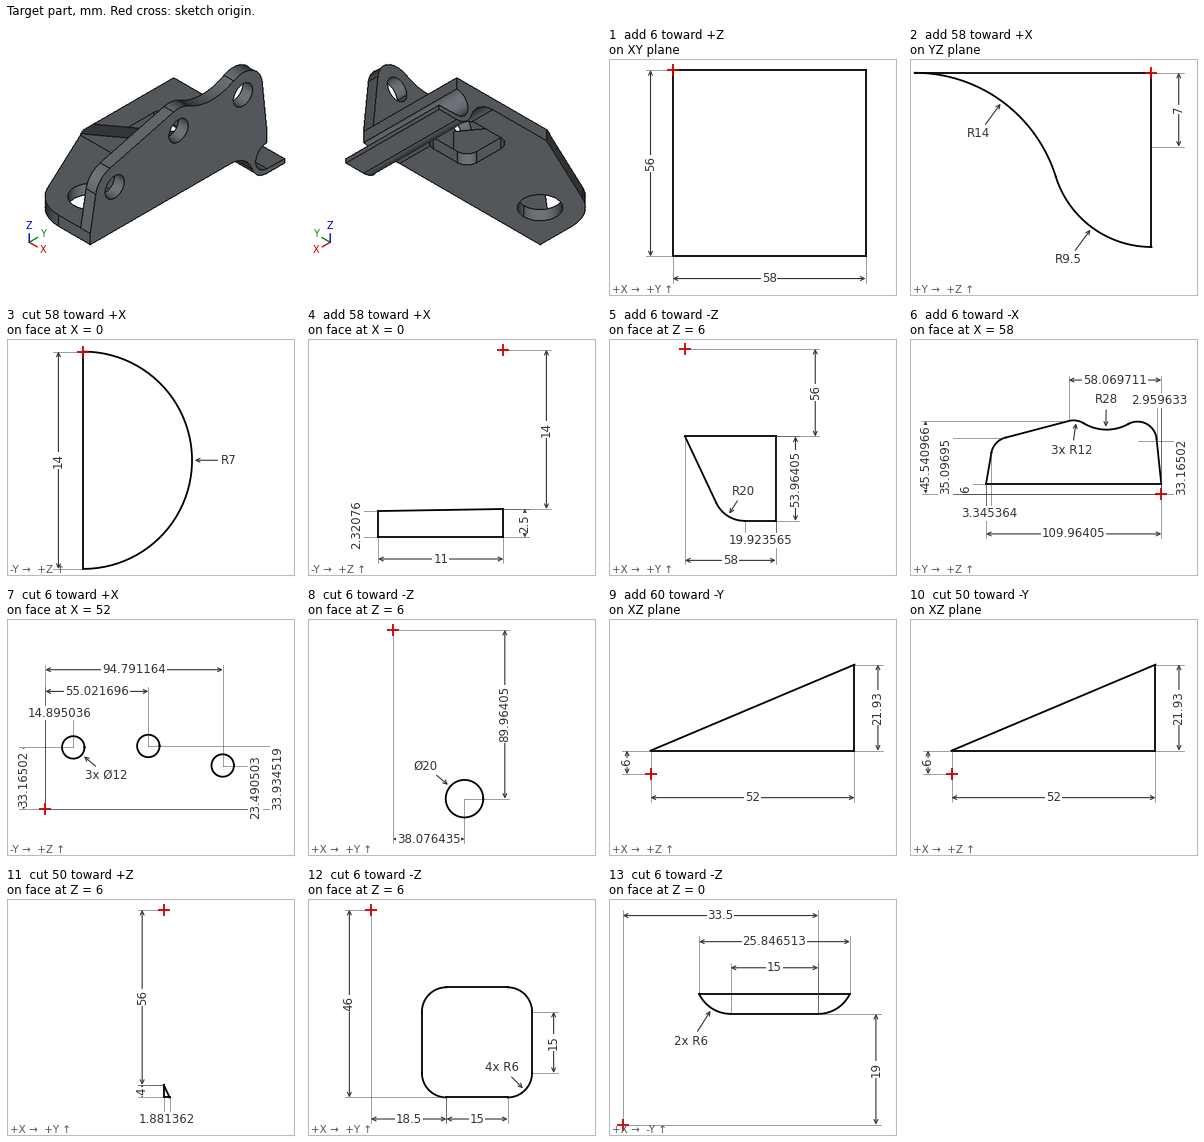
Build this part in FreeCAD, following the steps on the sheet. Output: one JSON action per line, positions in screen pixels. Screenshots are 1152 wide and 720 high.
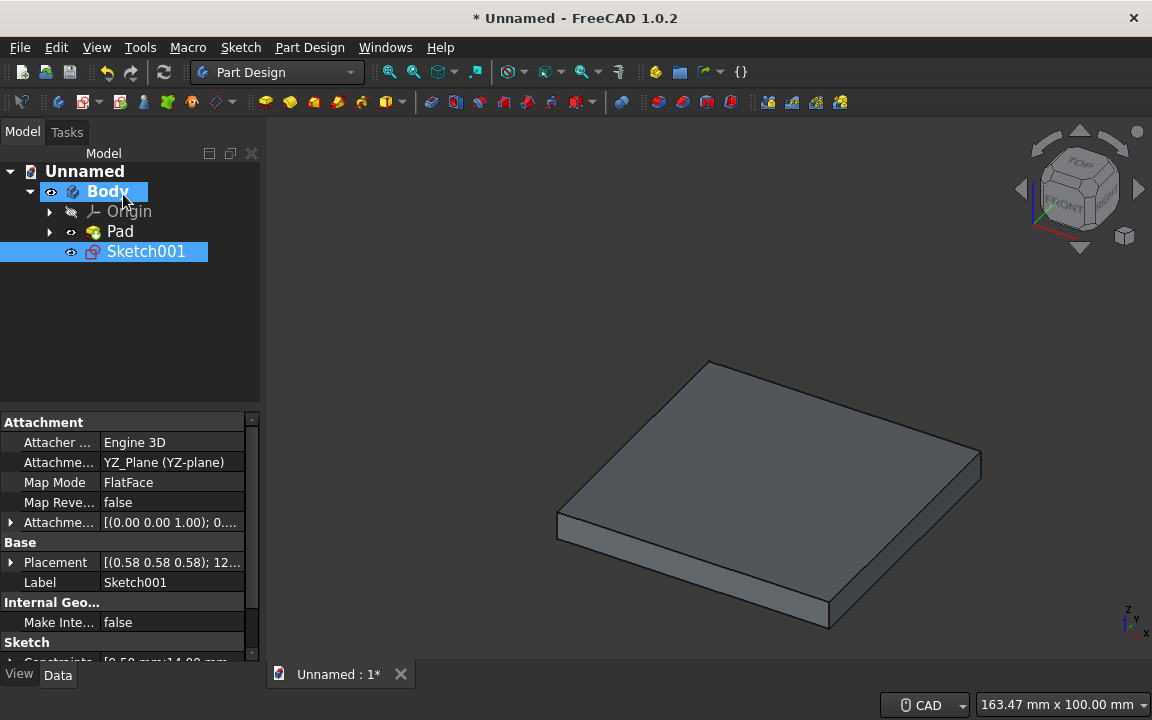
{"action": "left_click", "coordinate": [266, 102]}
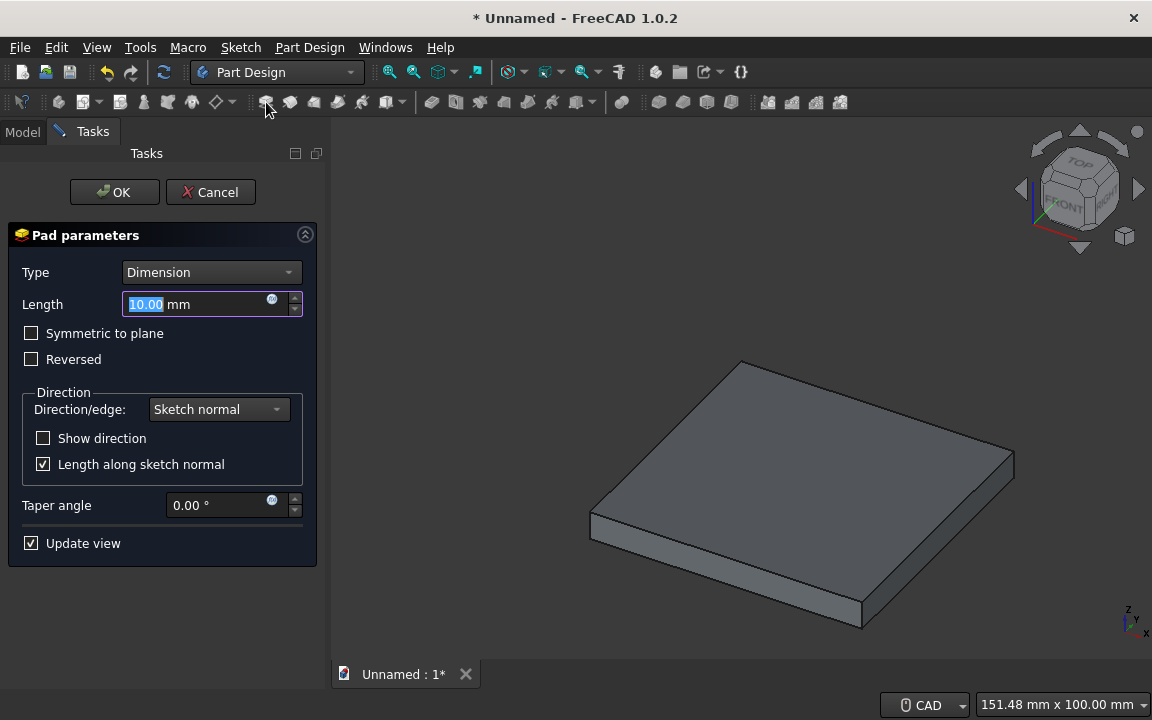
{"action": "type", "text": "58"}
{"action": "key", "text": "Tab"}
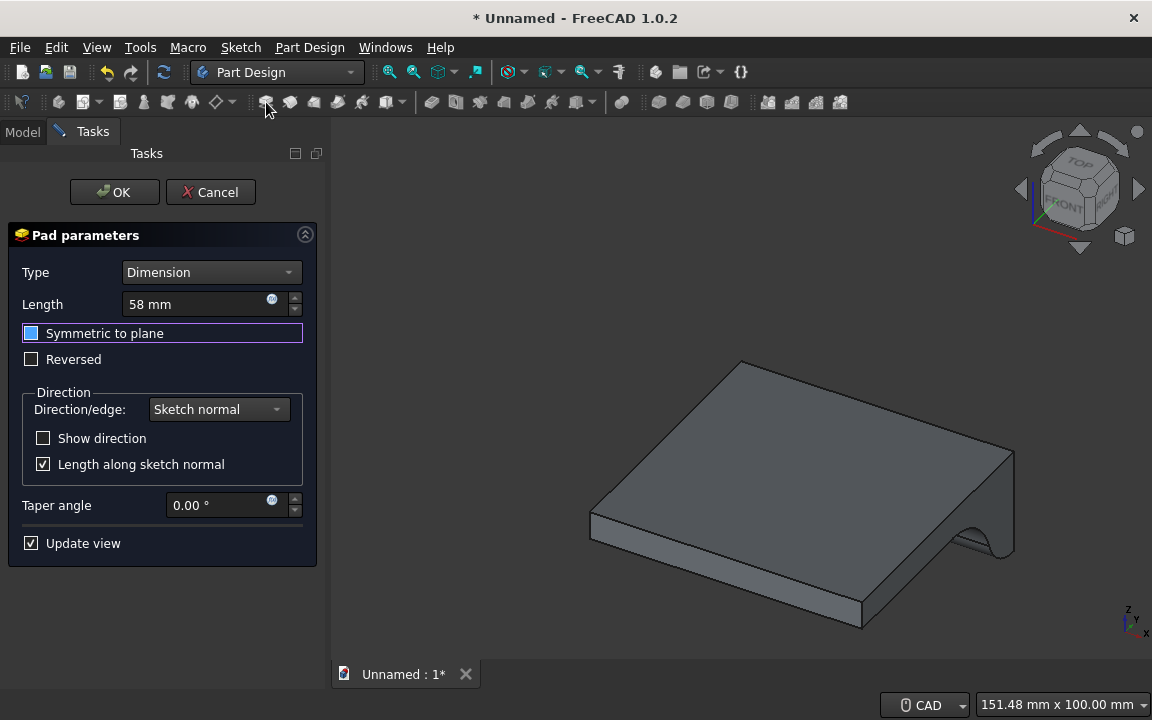
{"action": "left_click", "coordinate": [115, 192]}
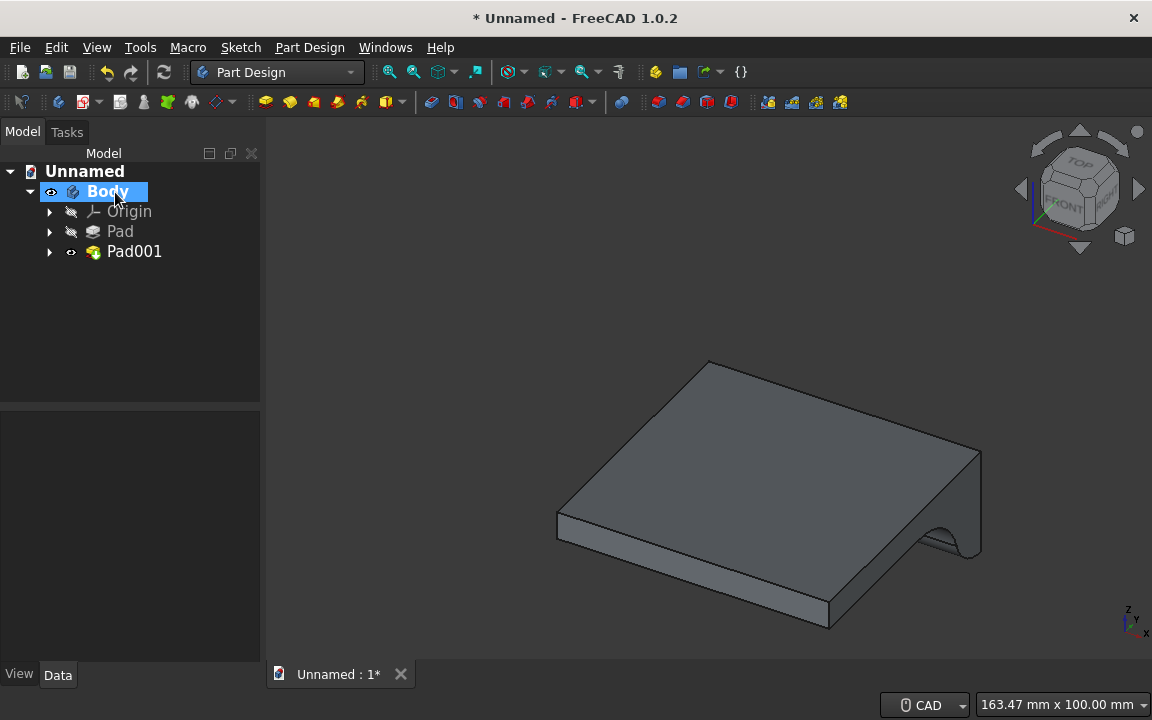
{"action": "left_click", "coordinate": [390, 72]}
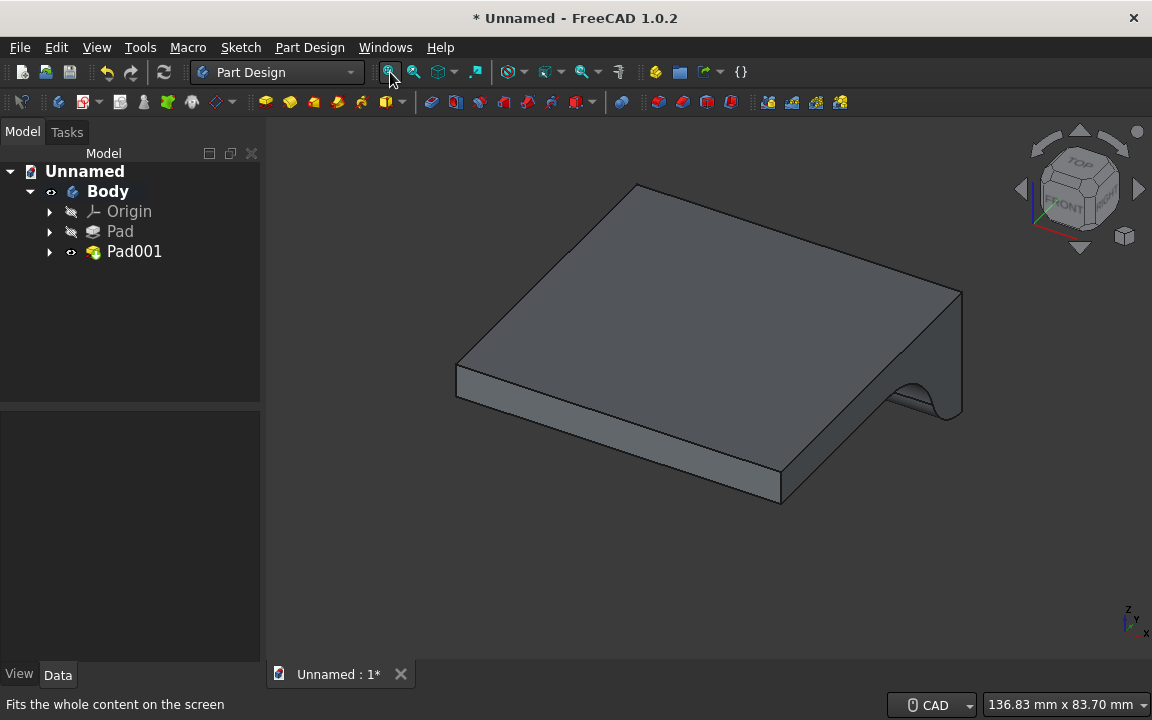
{"action": "key", "text": "6"}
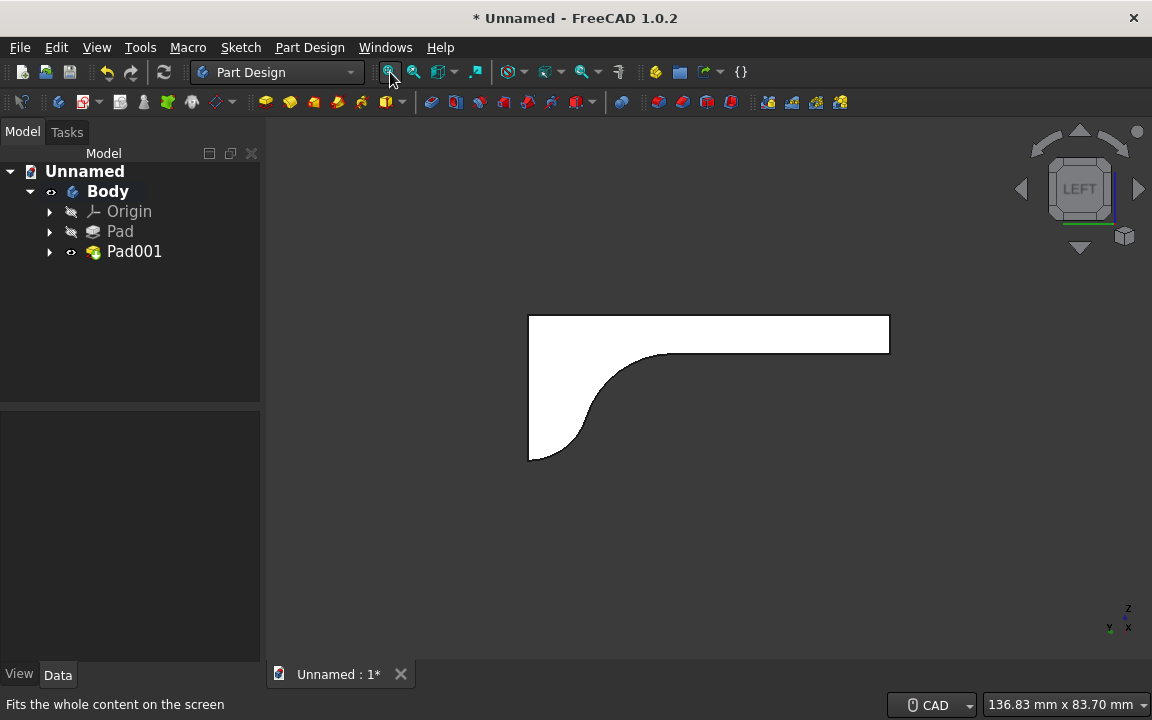
{"action": "left_click", "coordinate": [390, 72]}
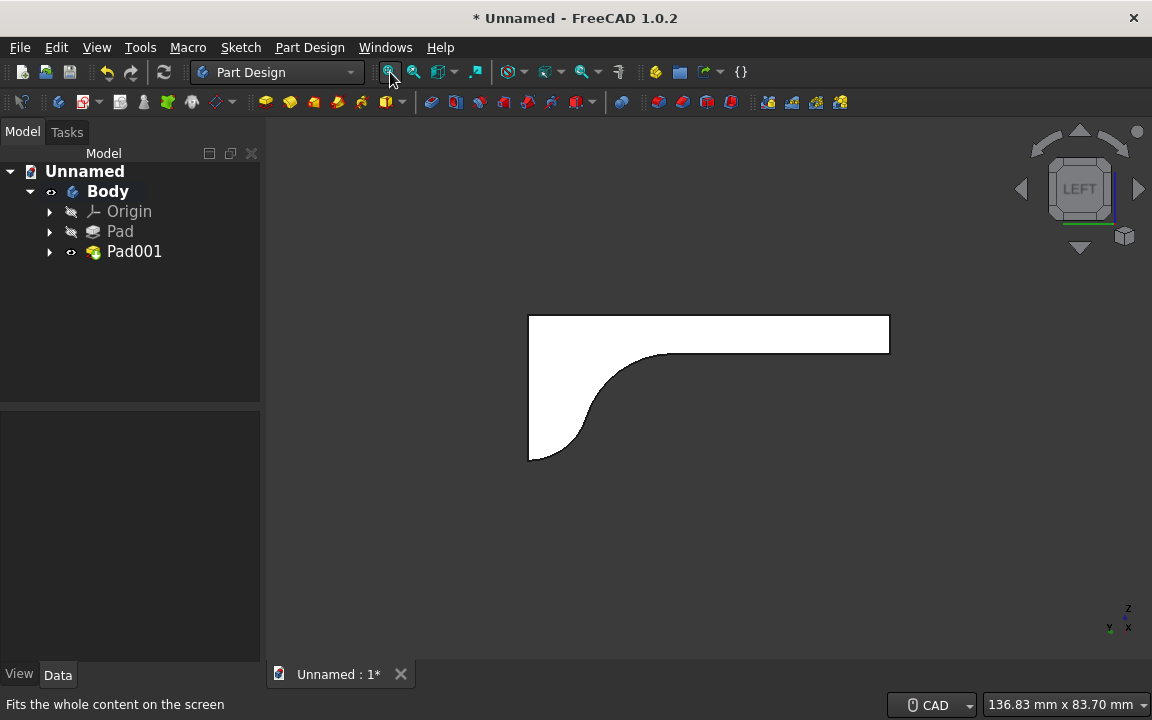
{"action": "left_click", "coordinate": [605, 345]}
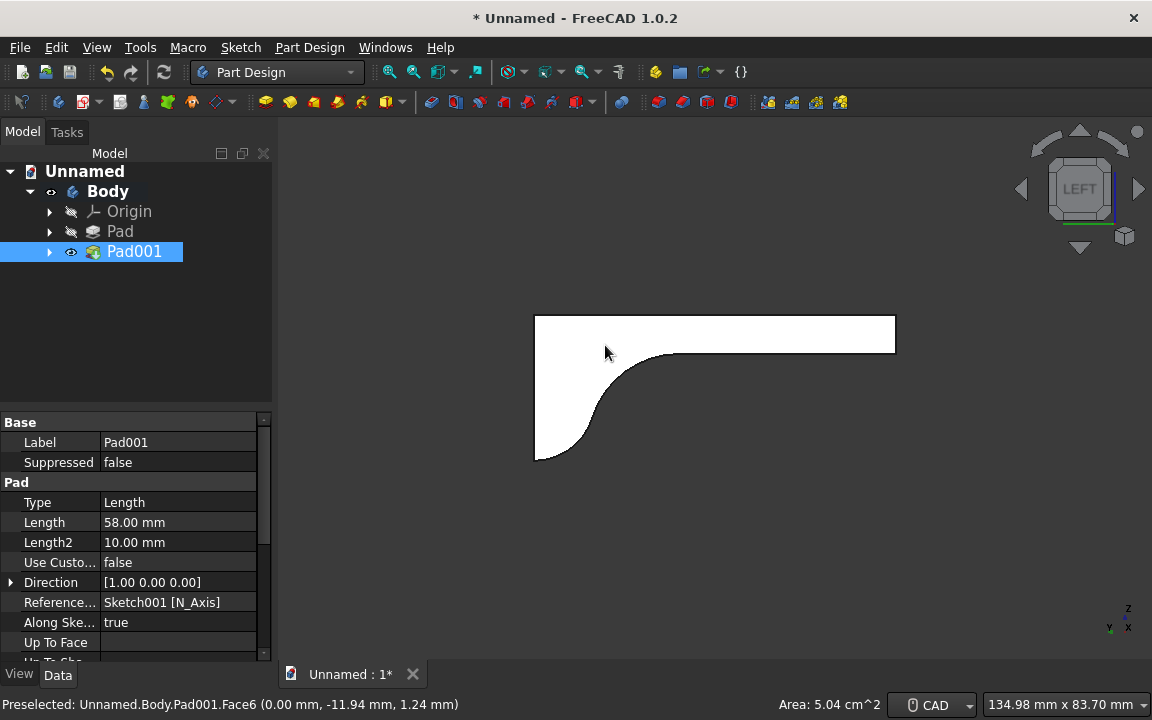
{"action": "left_click", "coordinate": [84, 102]}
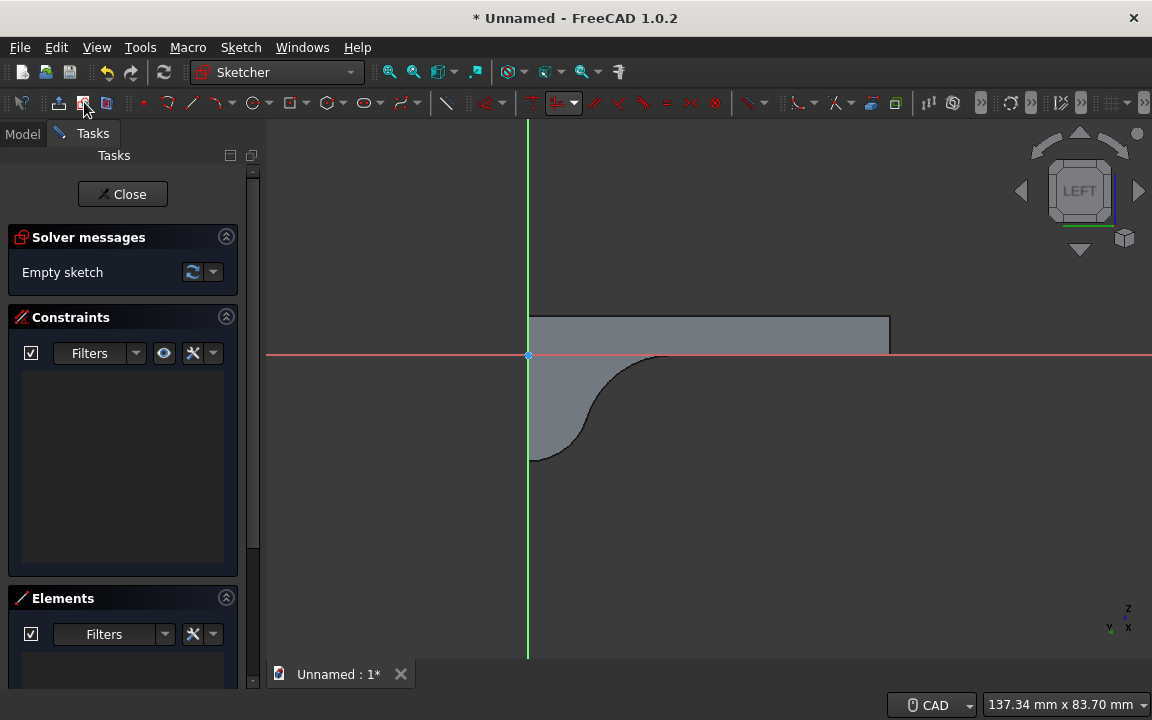
{"action": "scroll", "coordinate": [522, 404], "scroll_direction": "up", "scroll_amount": 7}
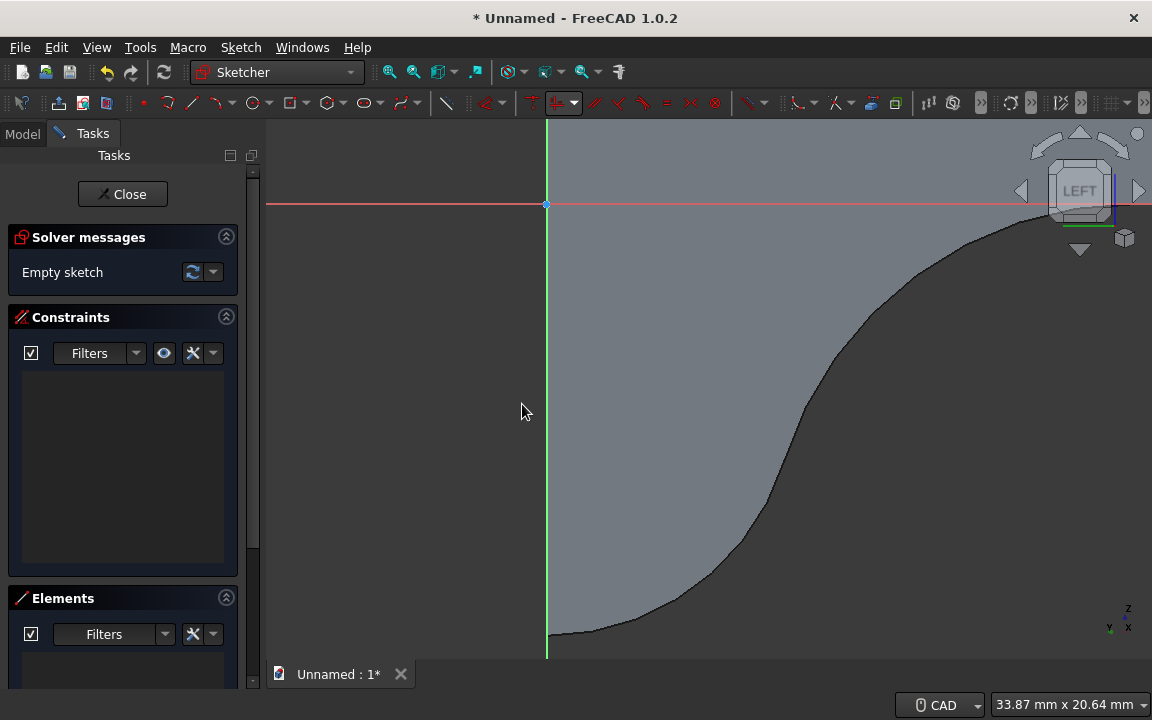
{"action": "left_click", "coordinate": [192, 104]}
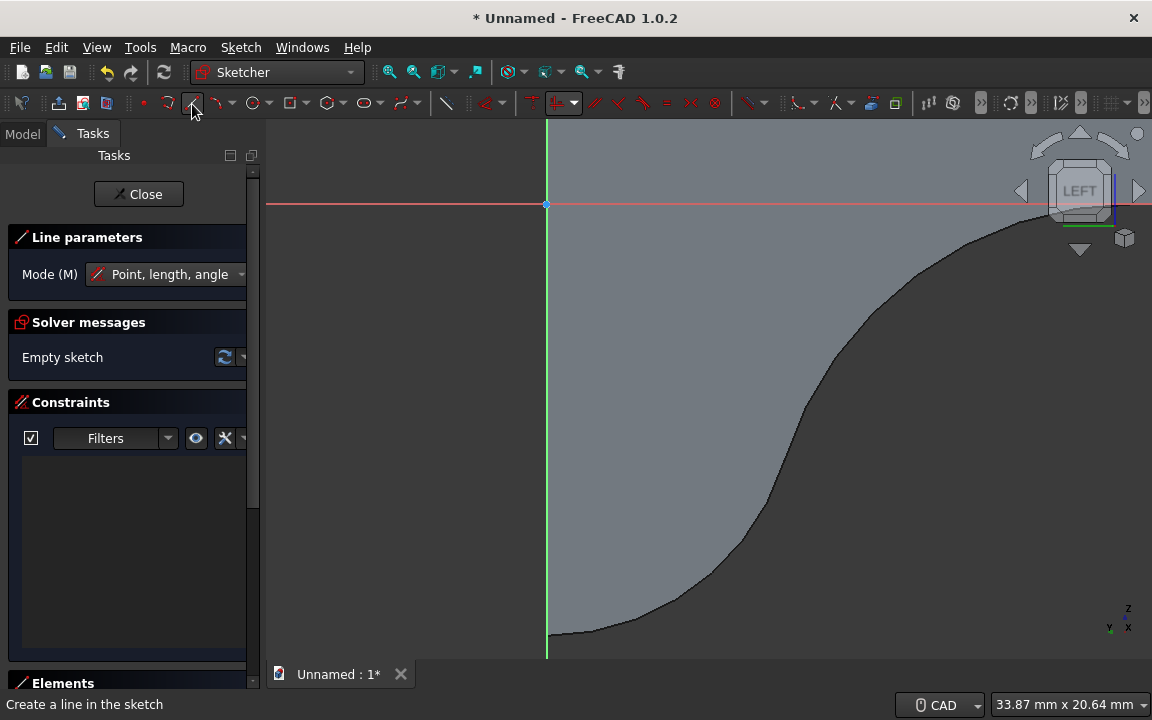
{"action": "left_click", "coordinate": [547, 204]}
{"action": "left_click", "coordinate": [556, 570]}